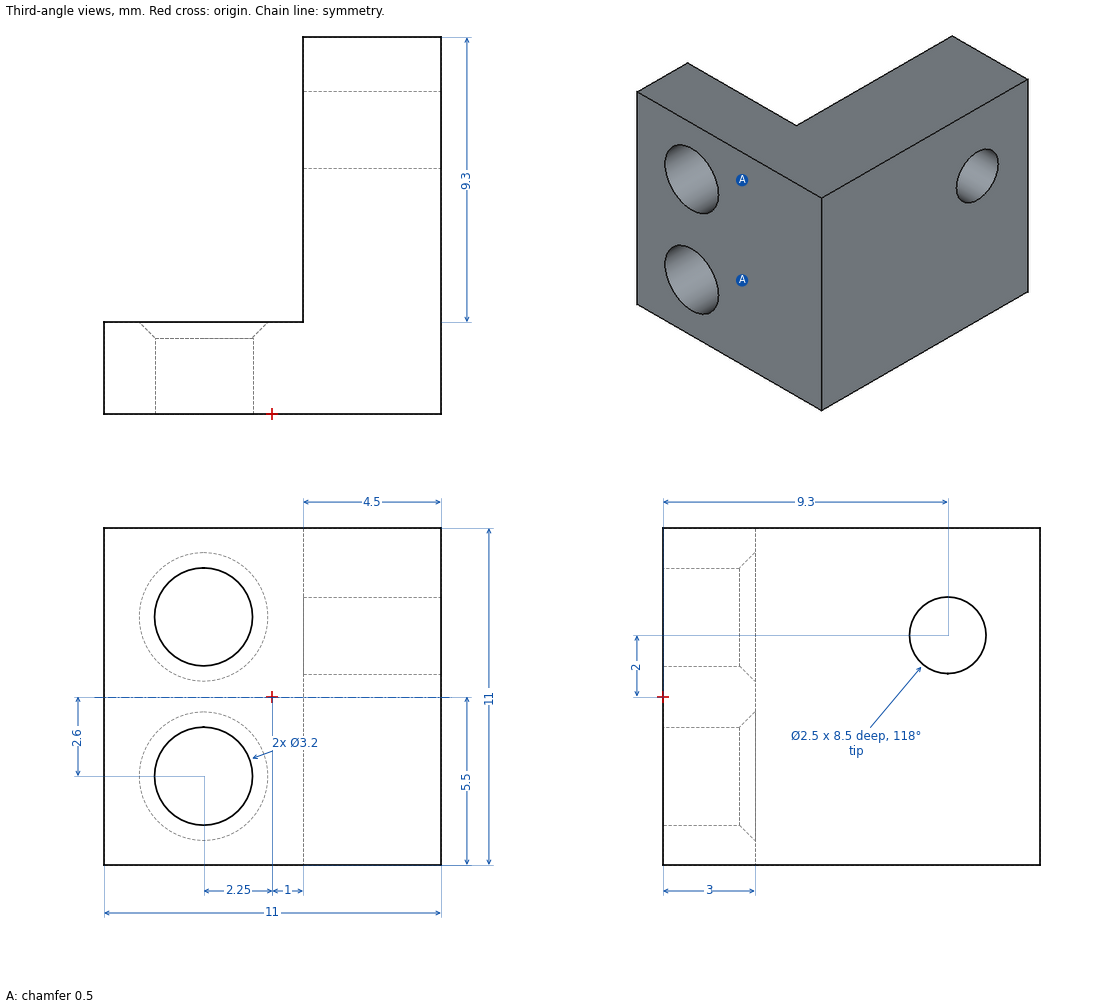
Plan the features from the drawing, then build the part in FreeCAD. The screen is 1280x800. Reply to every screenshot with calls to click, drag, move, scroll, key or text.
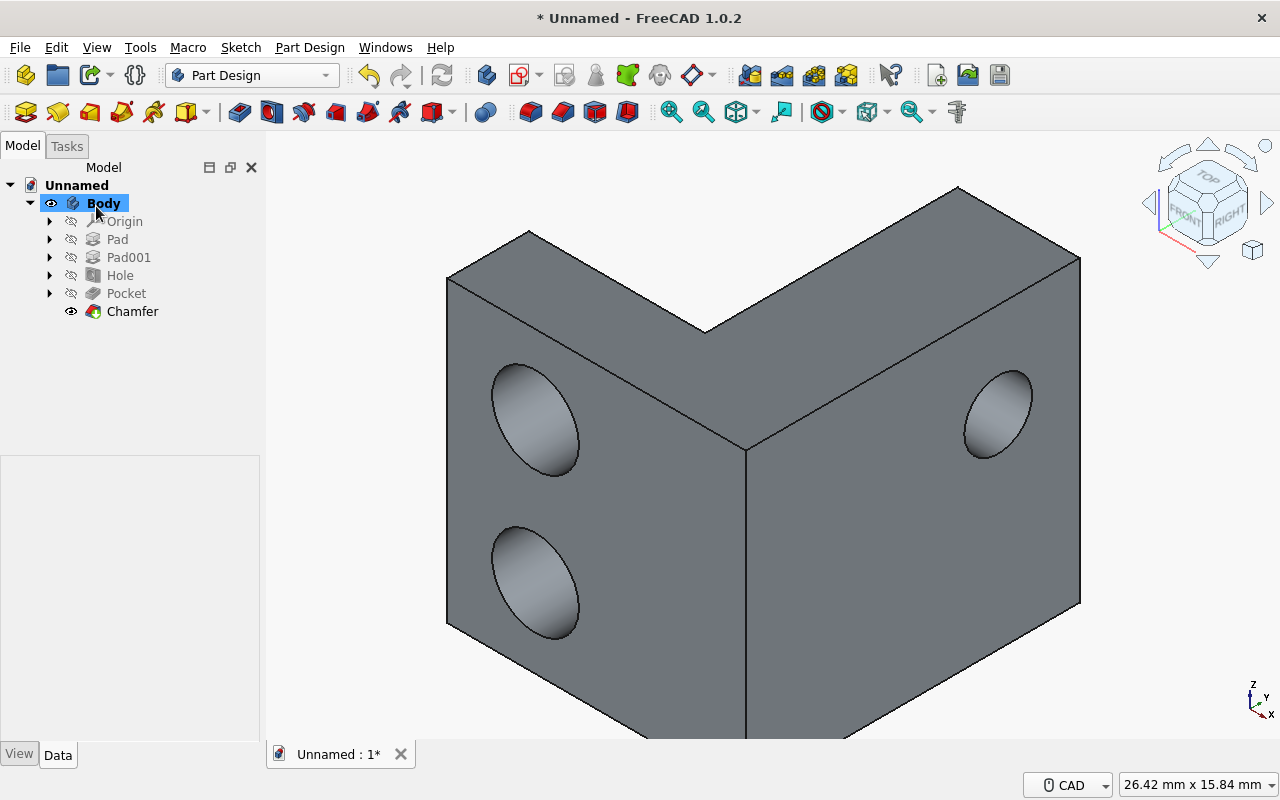
click(672, 112)